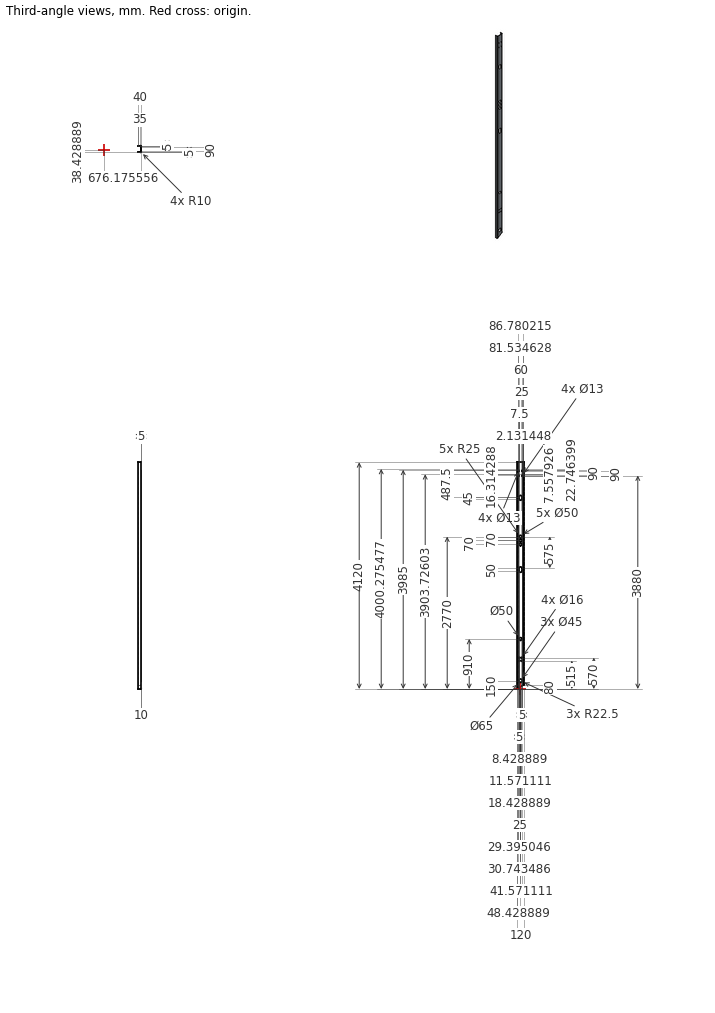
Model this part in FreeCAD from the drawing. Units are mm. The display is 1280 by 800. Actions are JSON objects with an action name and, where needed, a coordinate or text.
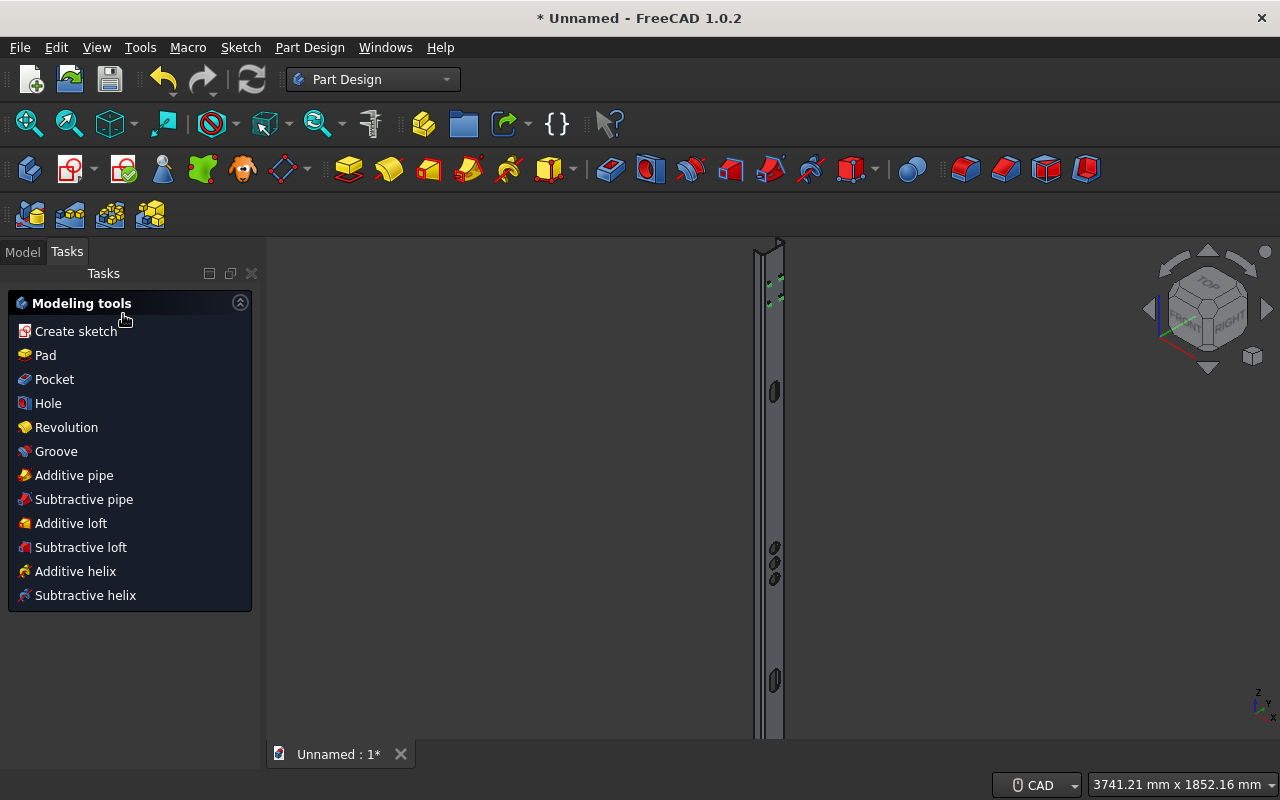
{"action": "left_click", "coordinate": [612, 170]}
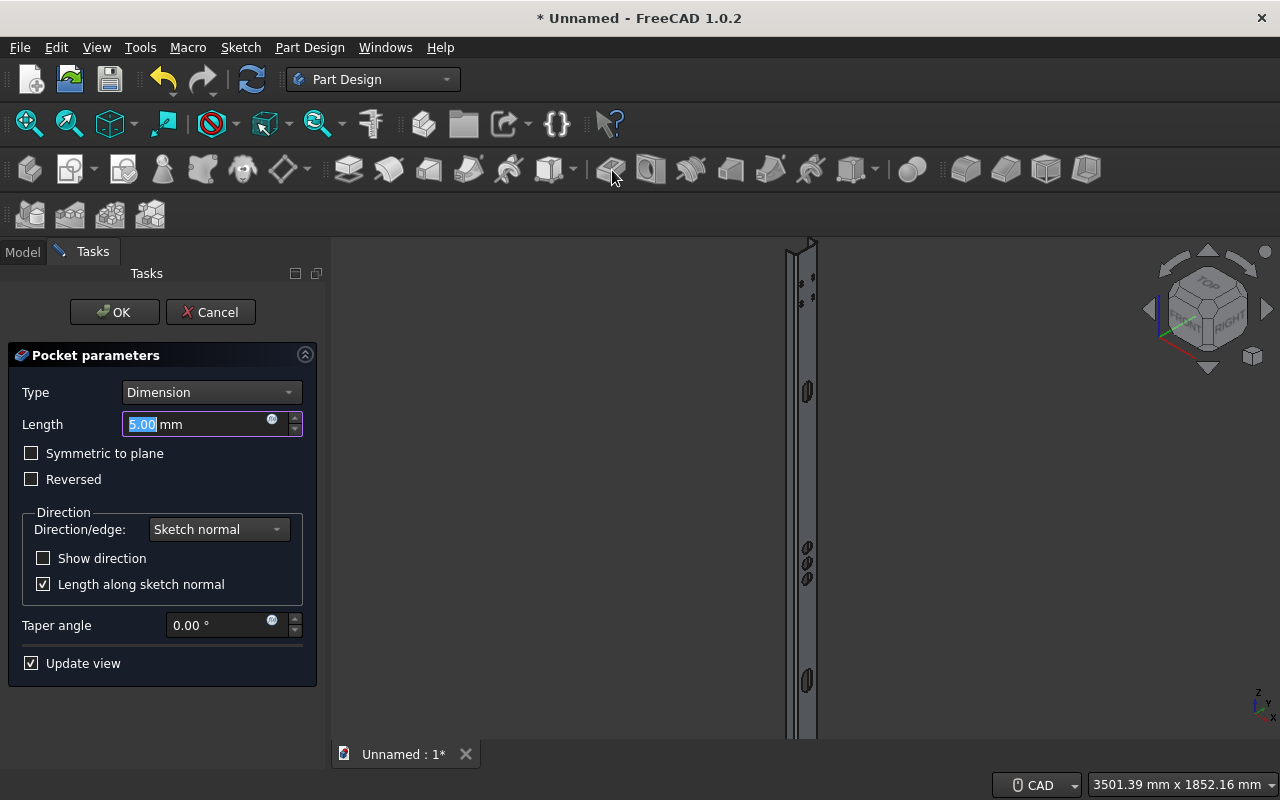
{"action": "type", "text": "10"}
{"action": "key", "text": "Tab"}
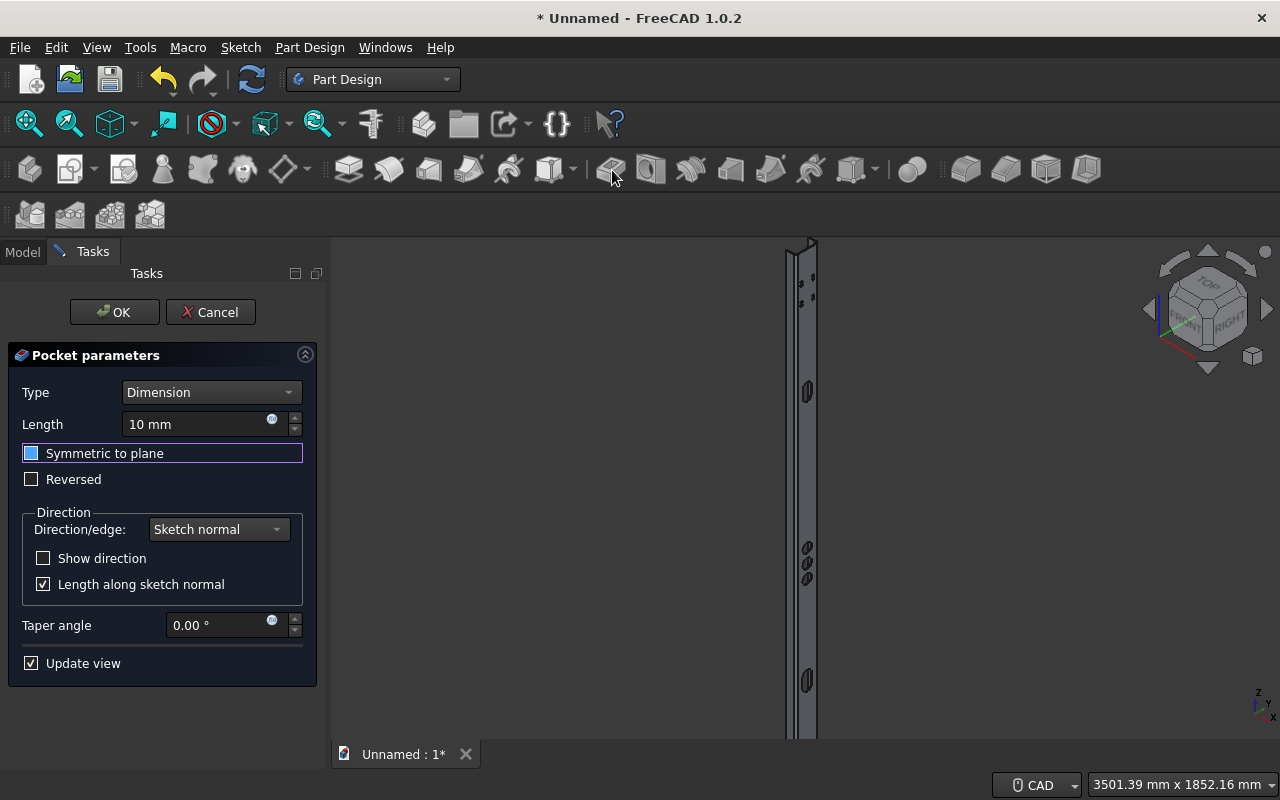
{"action": "left_click", "coordinate": [115, 312]}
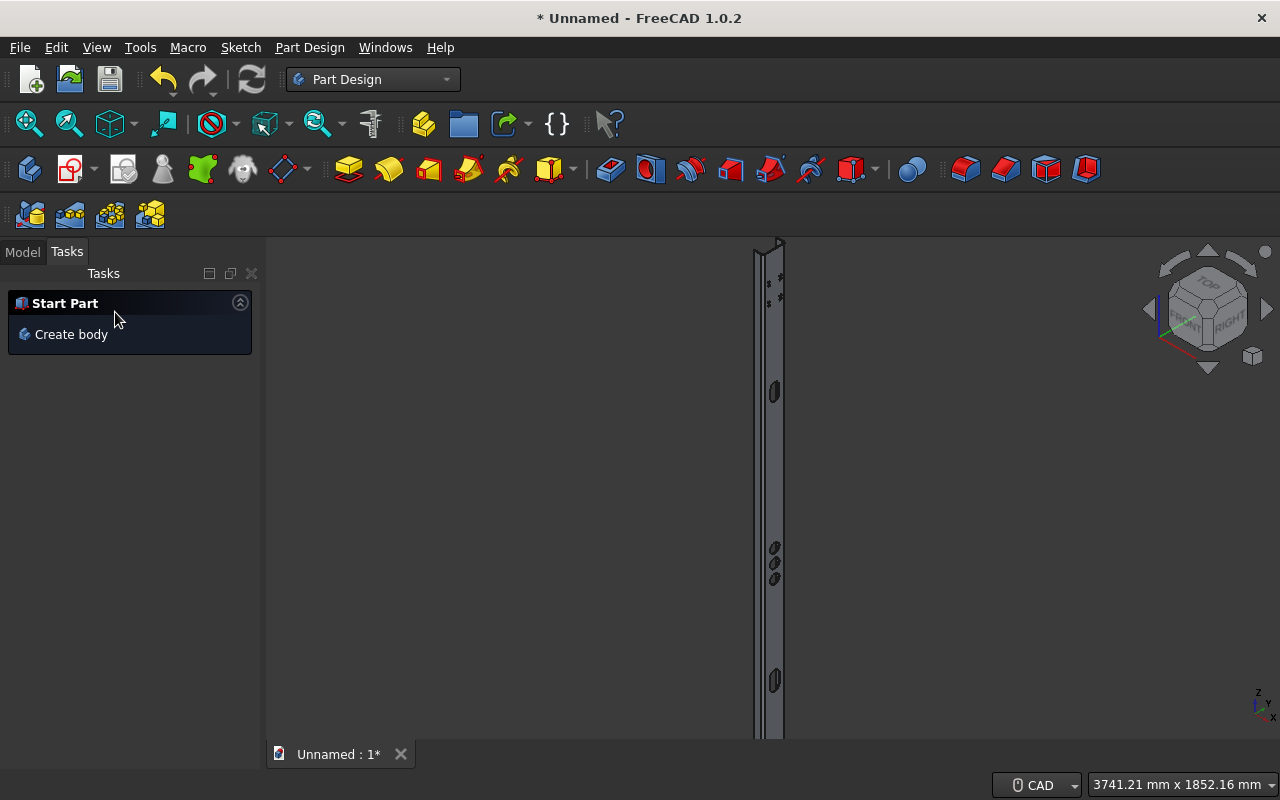
{"action": "left_click", "coordinate": [30, 124]}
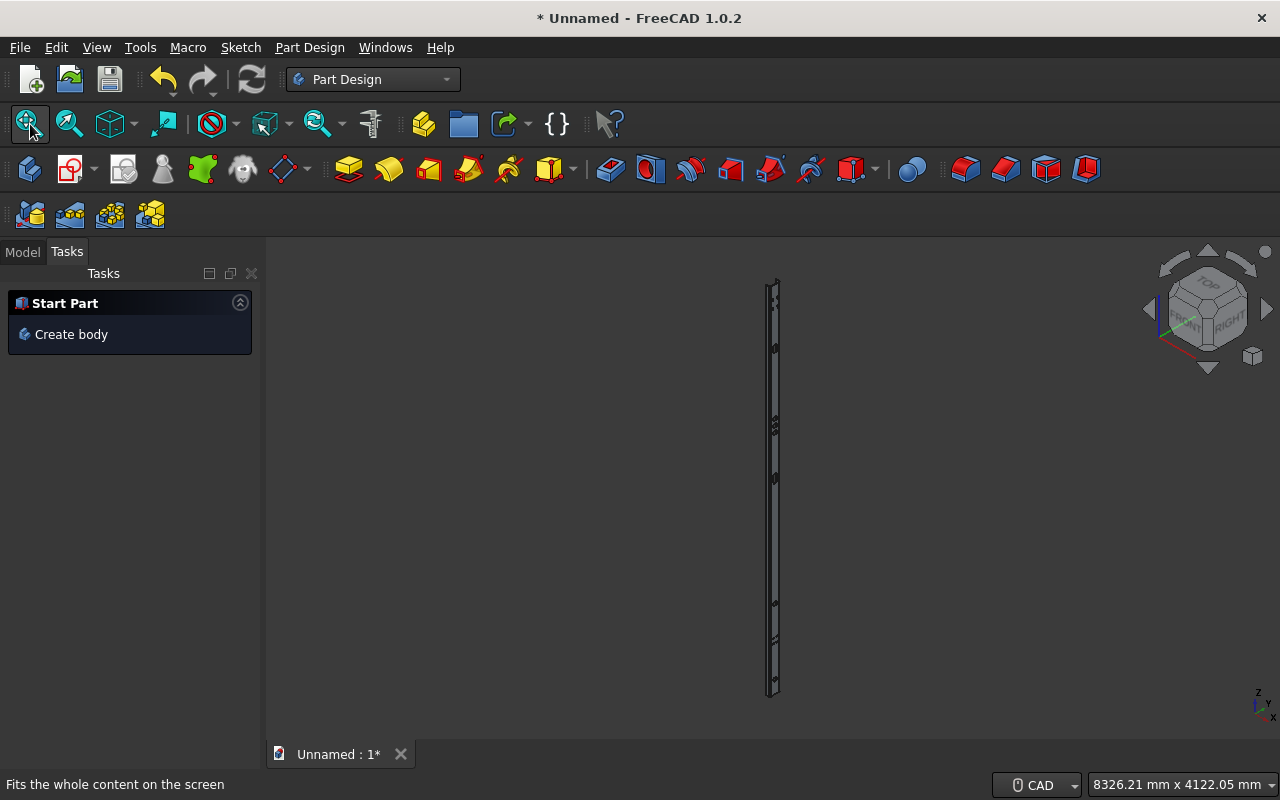
{"action": "scroll", "coordinate": [775, 313], "scroll_direction": "up", "scroll_amount": 4}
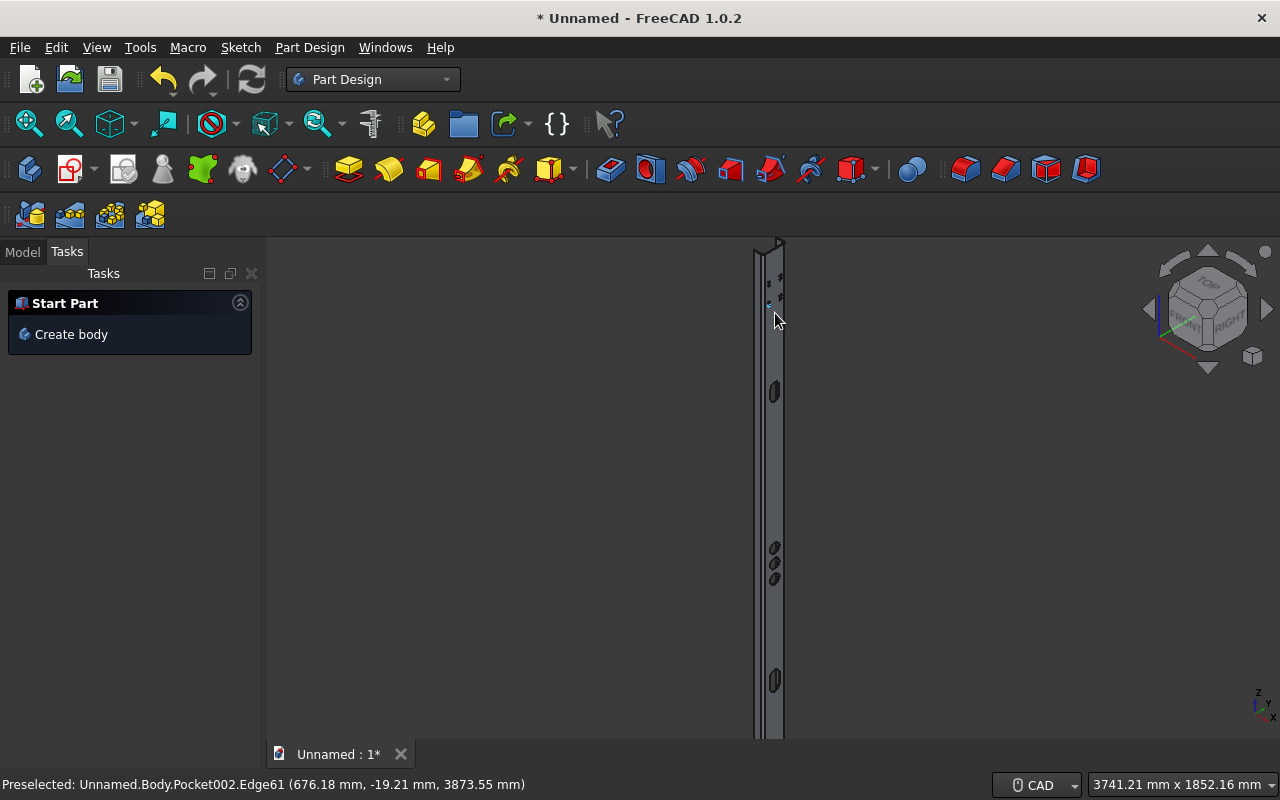
{"action": "left_click", "coordinate": [775, 444]}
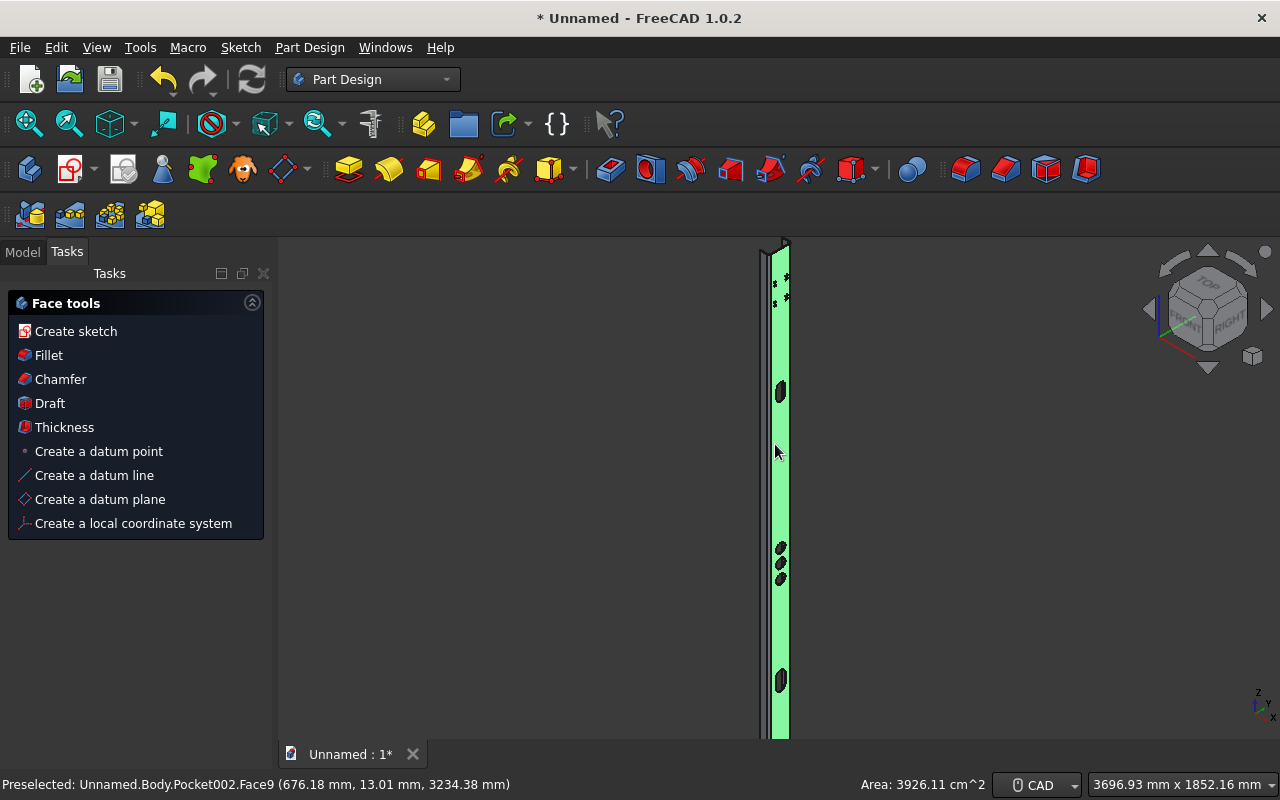
{"action": "left_click", "coordinate": [70, 170]}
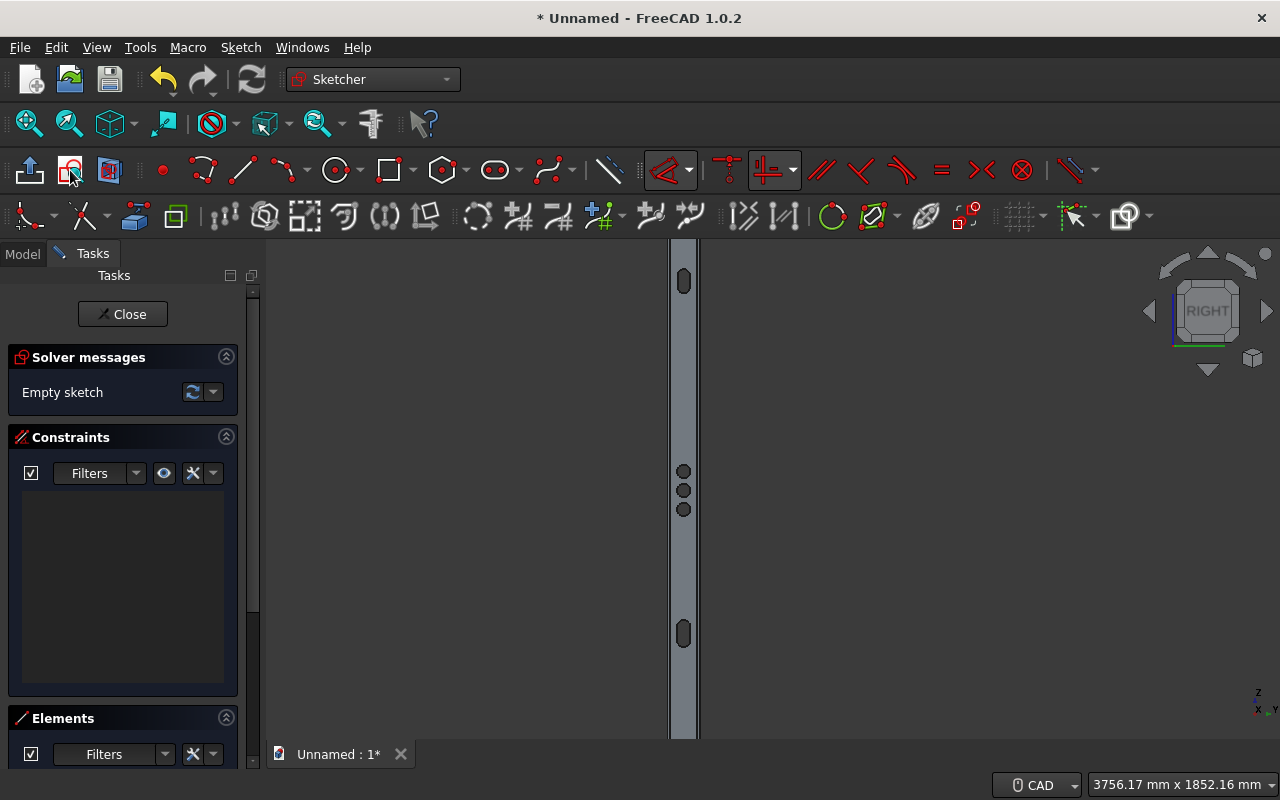
{"action": "scroll", "coordinate": [704, 489], "scroll_direction": "down", "scroll_amount": 5}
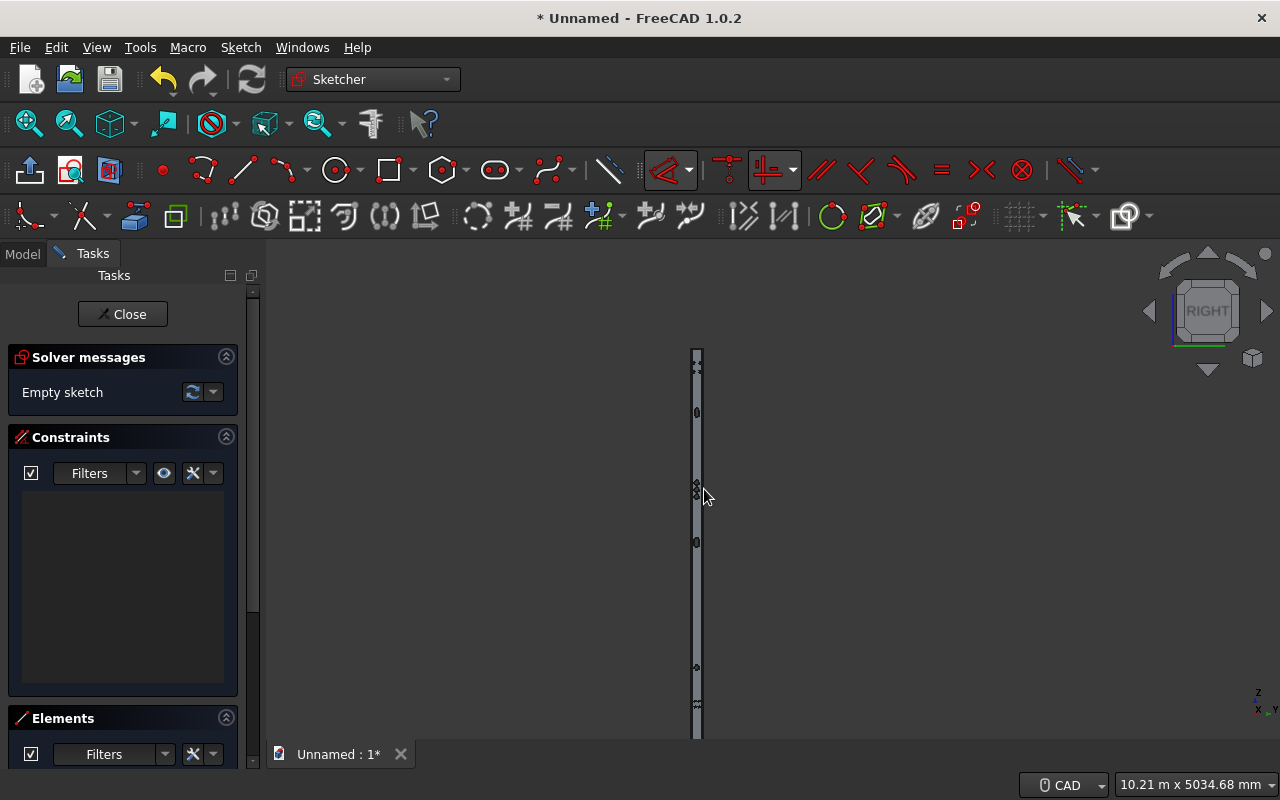
{"action": "scroll", "coordinate": [697, 360], "scroll_direction": "up", "scroll_amount": 15}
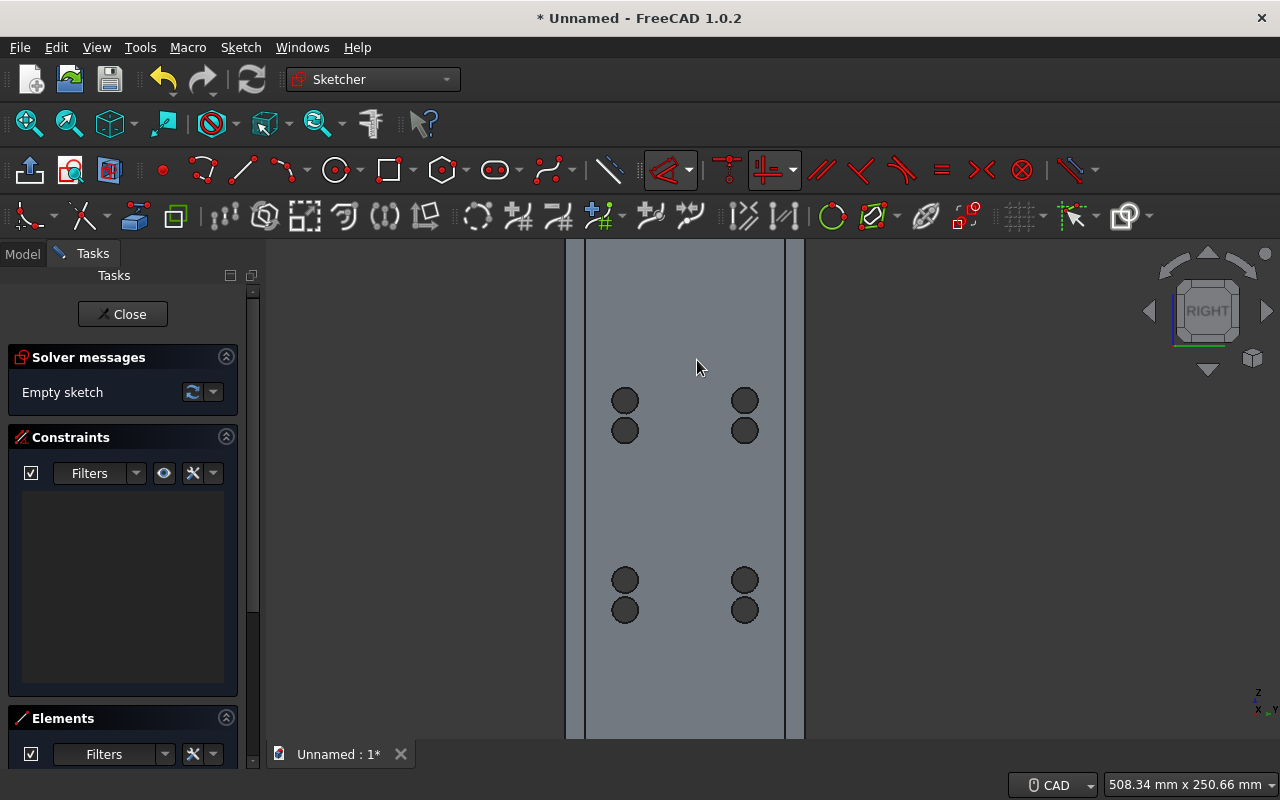
{"action": "scroll", "coordinate": [652, 470], "scroll_direction": "up", "scroll_amount": 2}